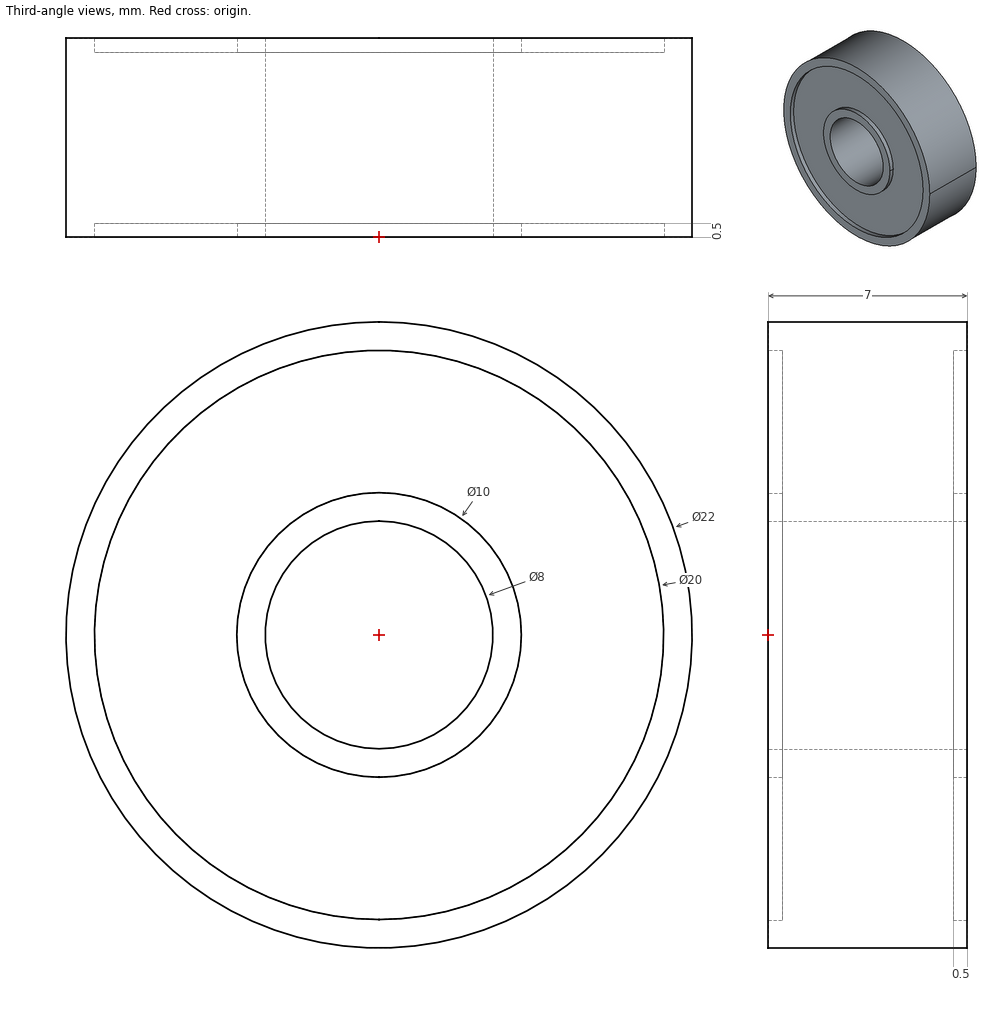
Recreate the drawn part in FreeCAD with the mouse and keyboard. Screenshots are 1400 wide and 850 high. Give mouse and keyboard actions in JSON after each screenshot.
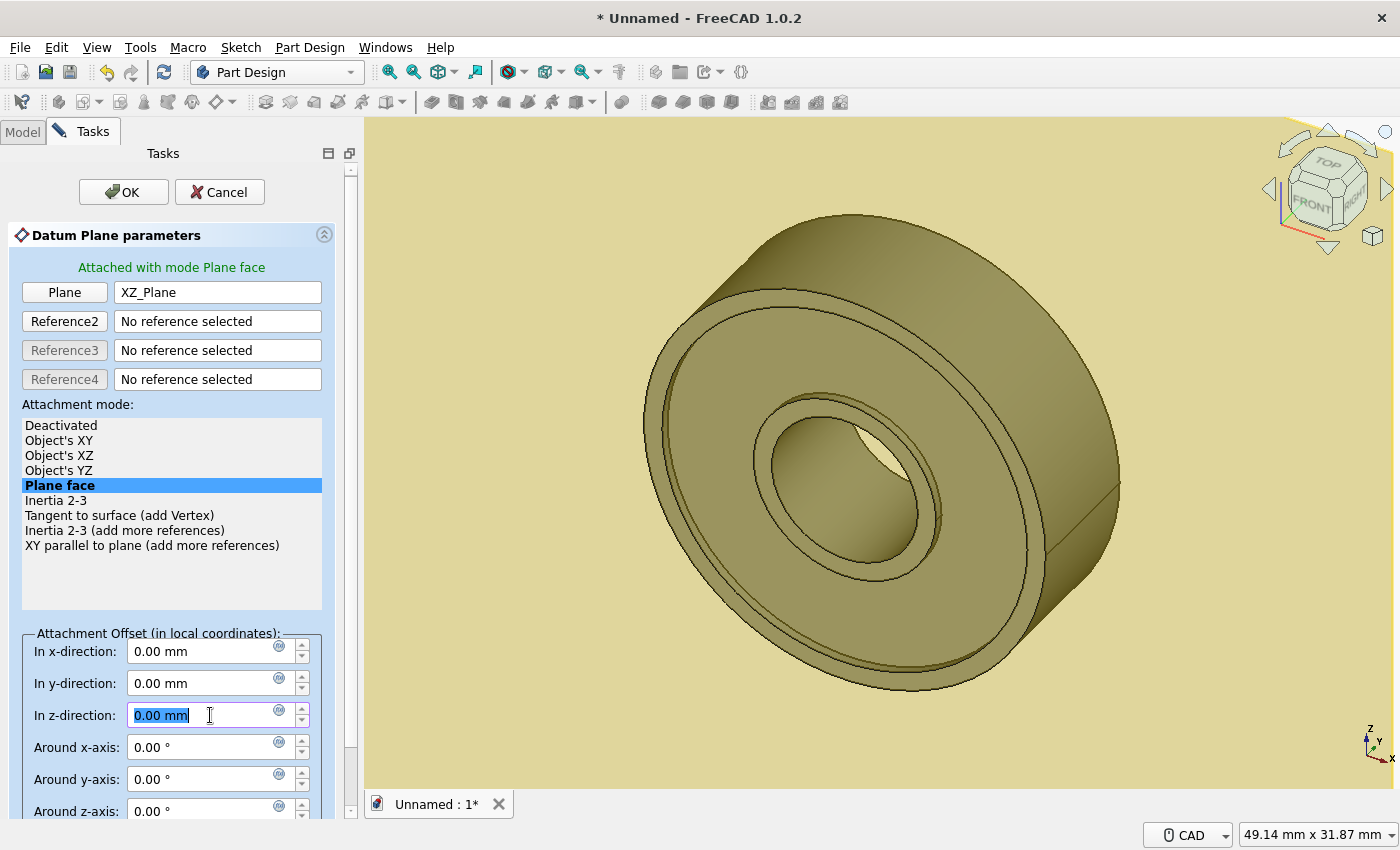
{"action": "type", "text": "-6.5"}
{"action": "key", "text": "Tab"}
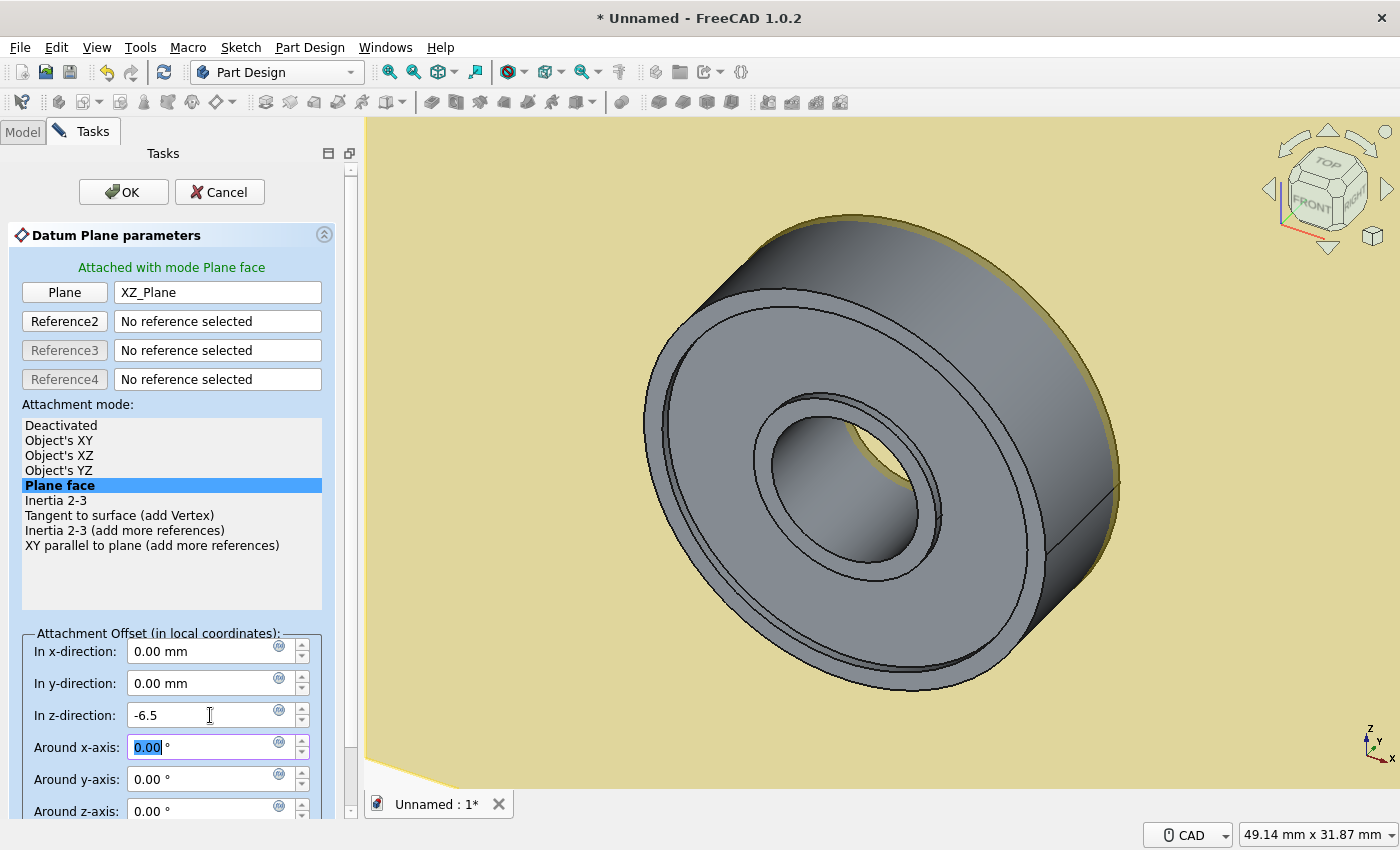
{"action": "left_click", "coordinate": [124, 192]}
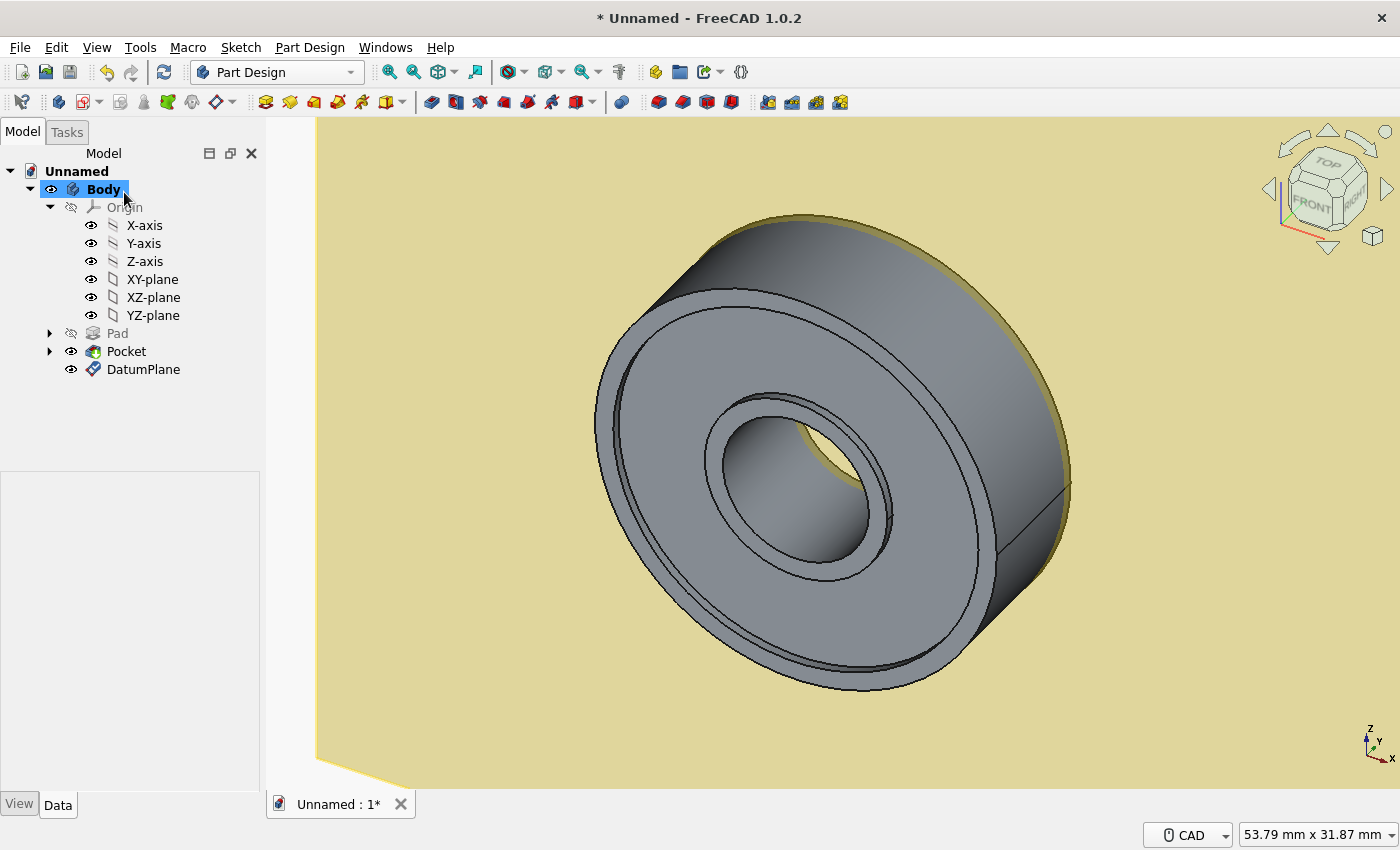
{"action": "left_click", "coordinate": [116, 369]}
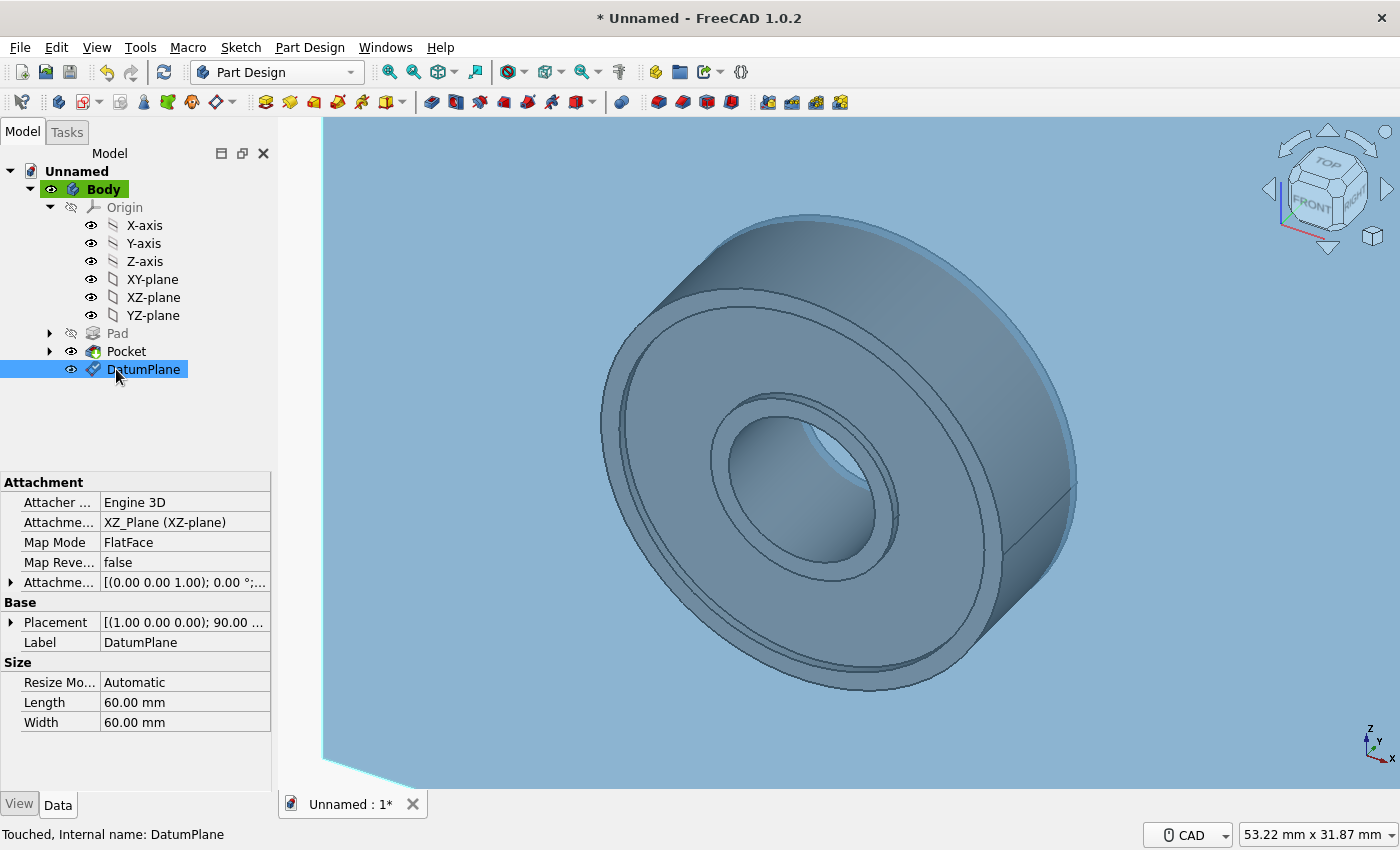
{"action": "left_click", "coordinate": [84, 102]}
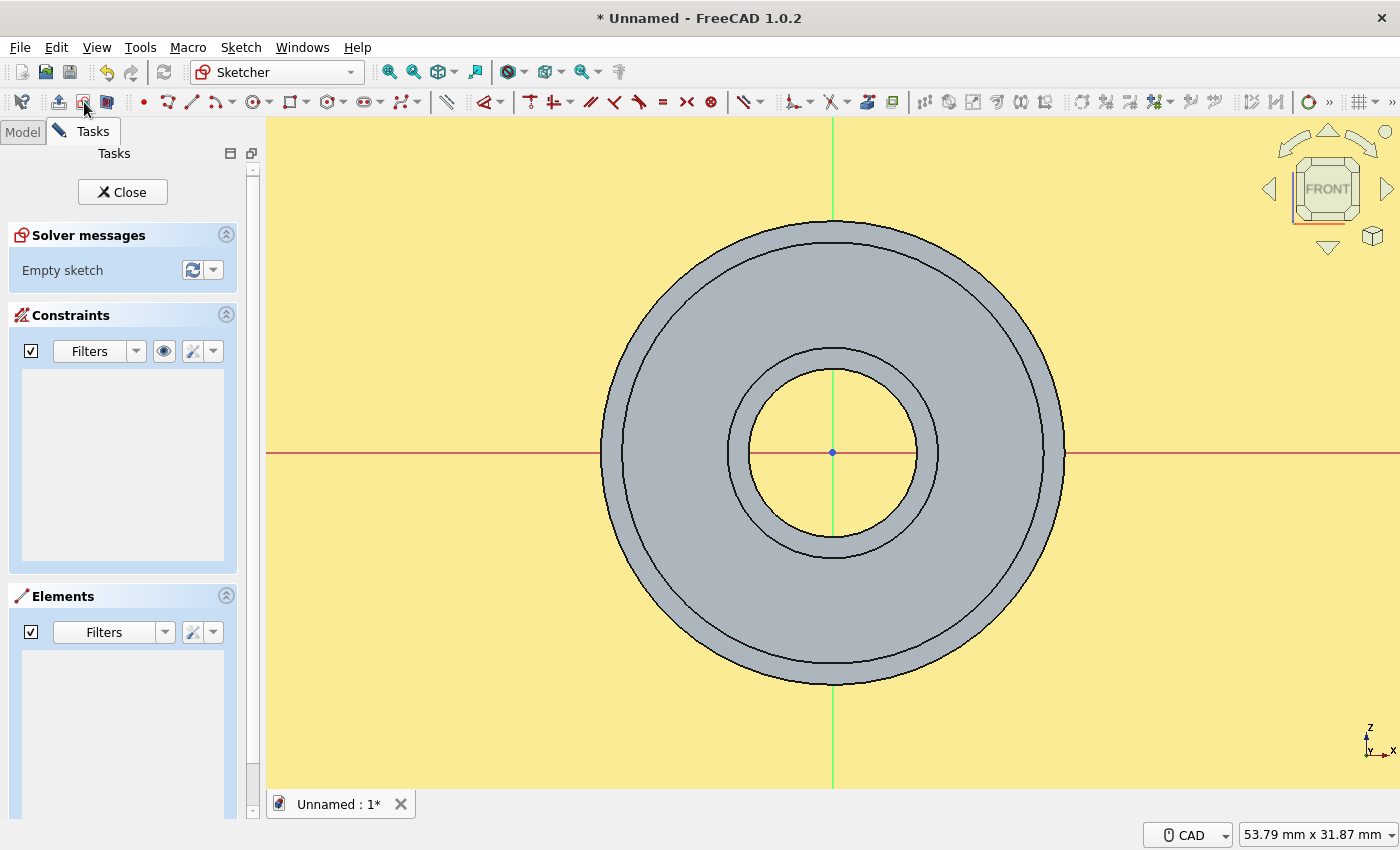
{"action": "left_click", "coordinate": [108, 102]}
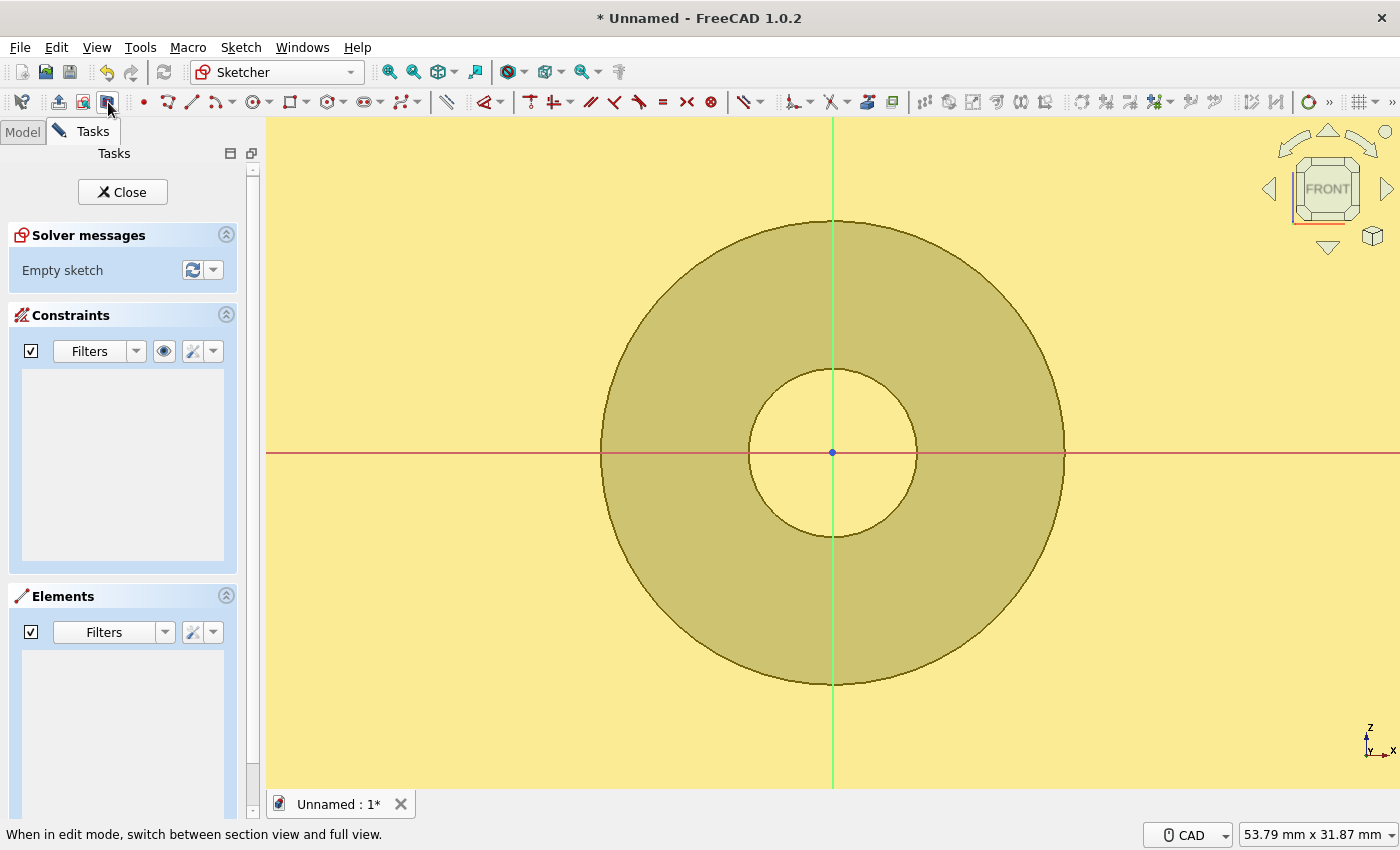
{"action": "left_click", "coordinate": [254, 102]}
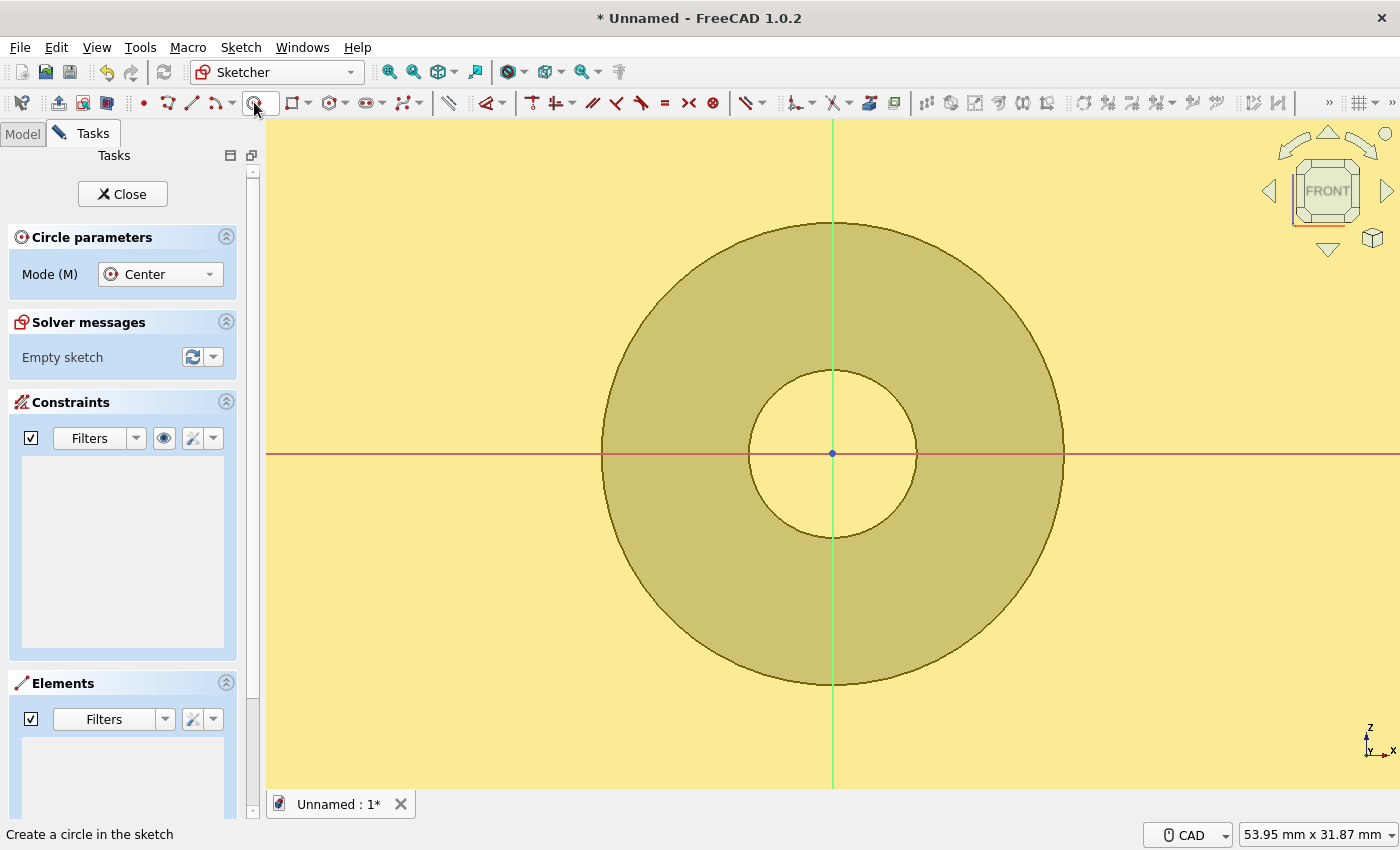
{"action": "left_click", "coordinate": [833, 454]}
{"action": "mouse_move", "coordinate": [981, 305]}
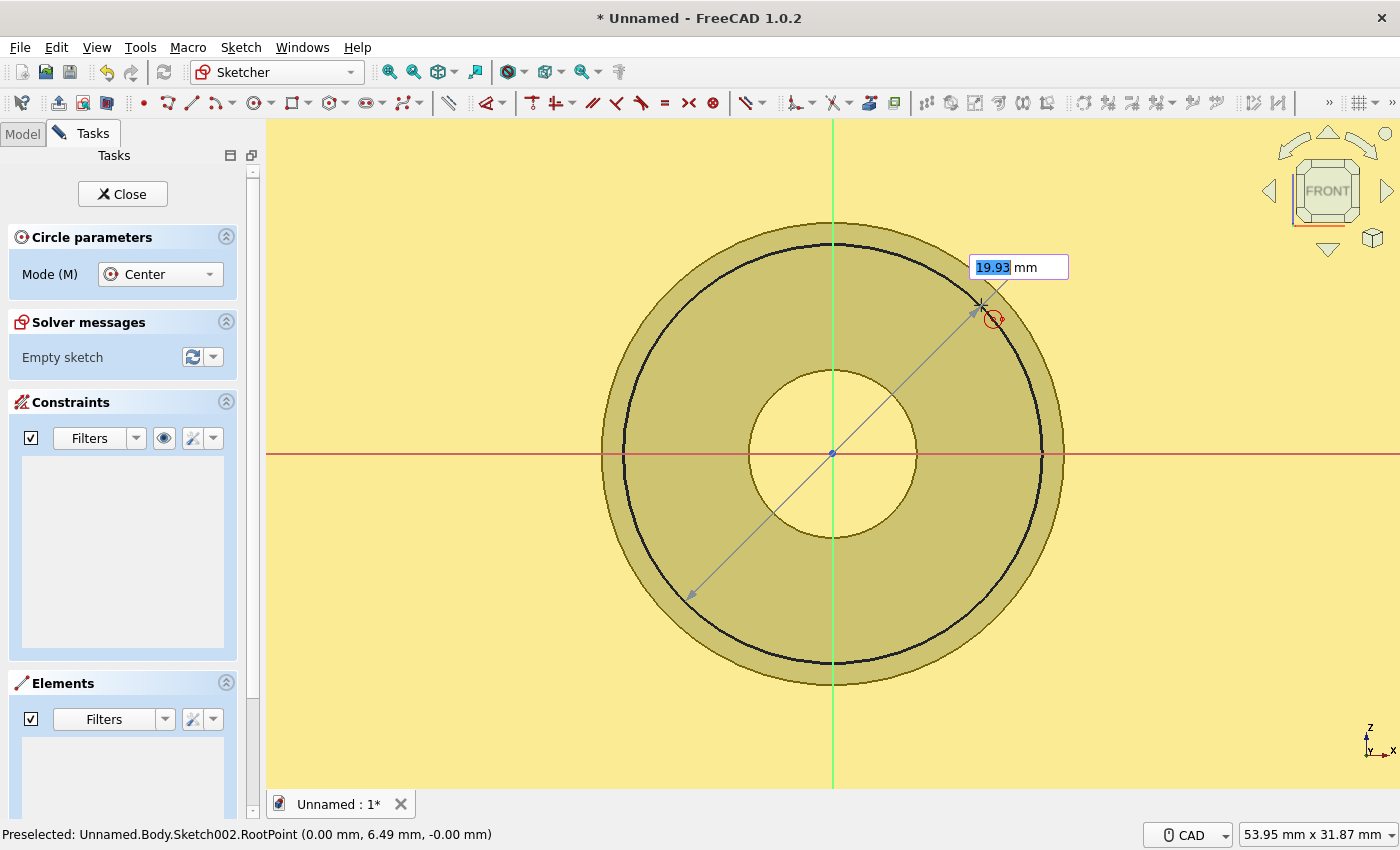
{"action": "type", "text": "20"}
{"action": "key", "text": "Return"}